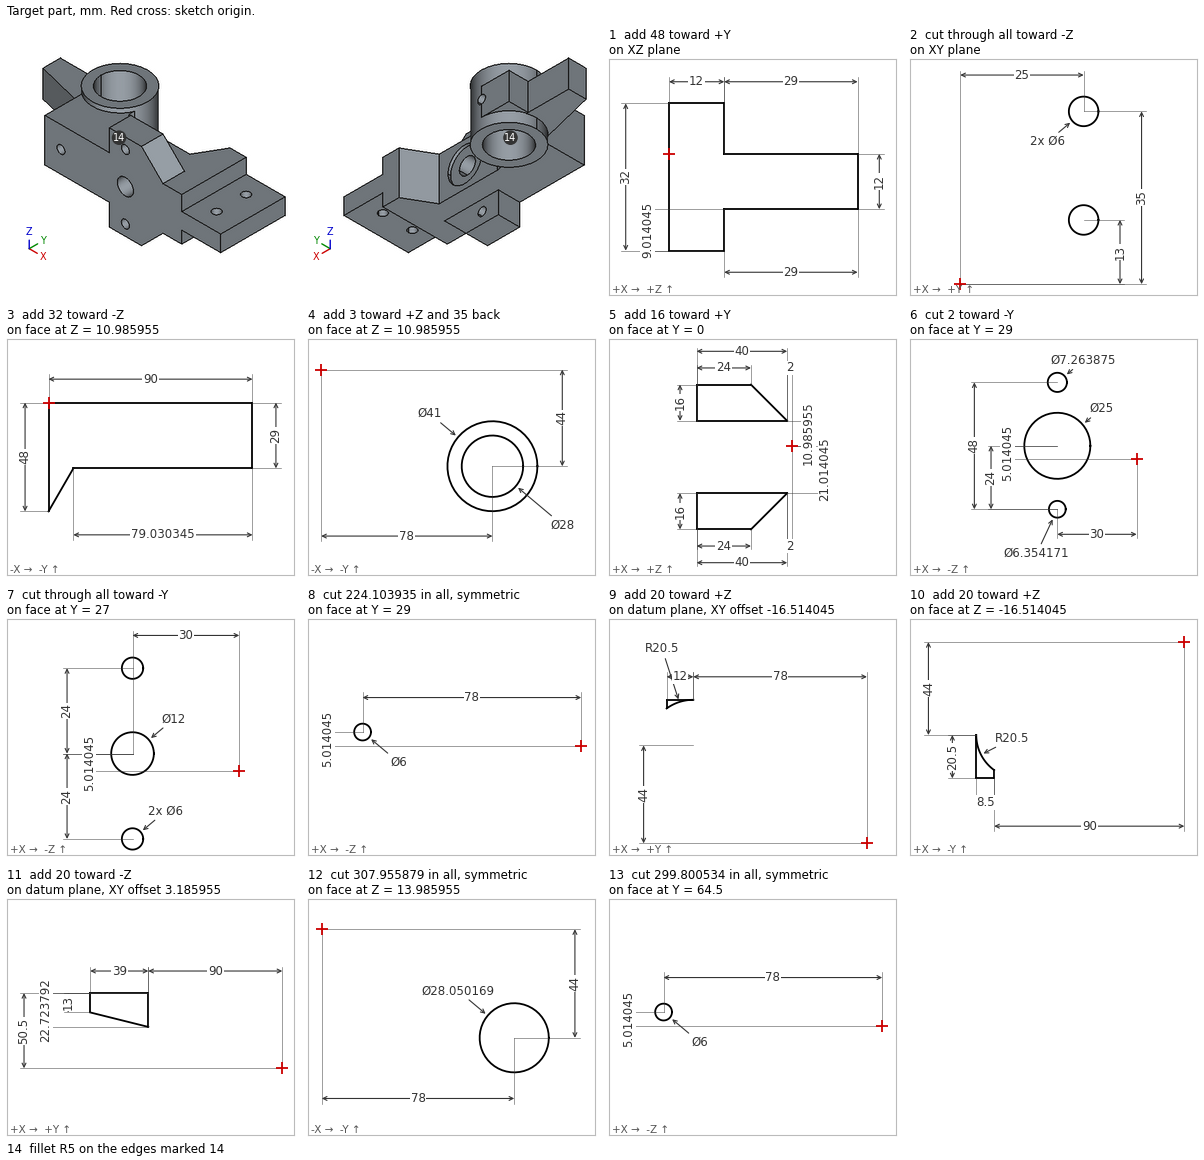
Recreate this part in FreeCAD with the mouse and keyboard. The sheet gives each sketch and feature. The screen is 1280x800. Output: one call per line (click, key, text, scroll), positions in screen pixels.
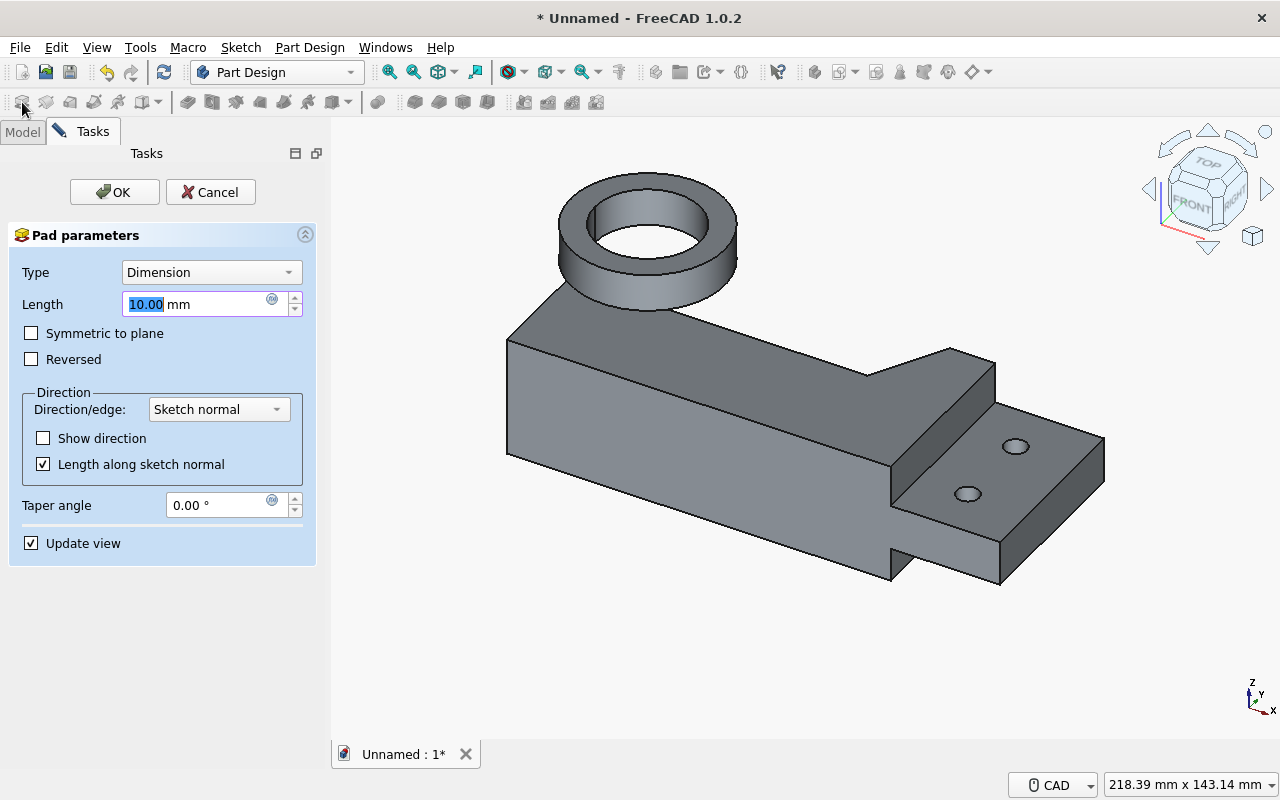
click(212, 272)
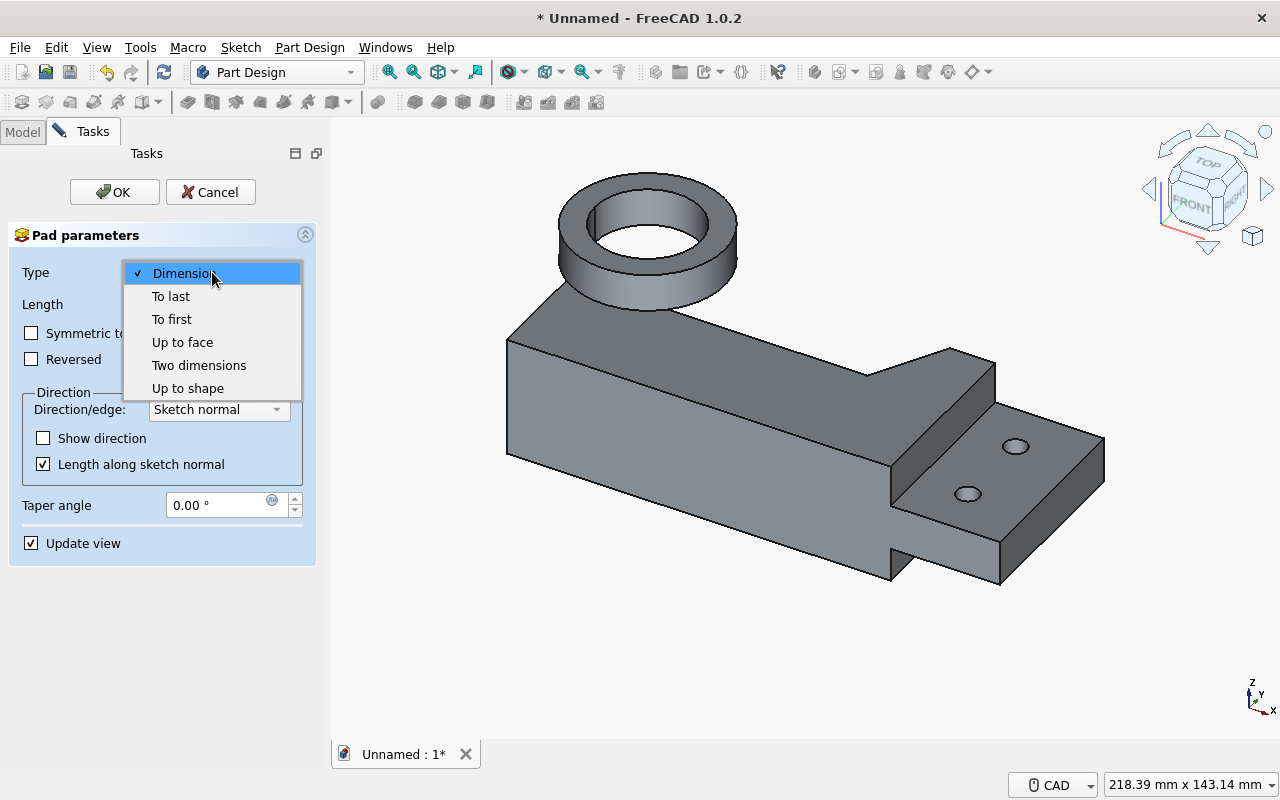
click(212, 366)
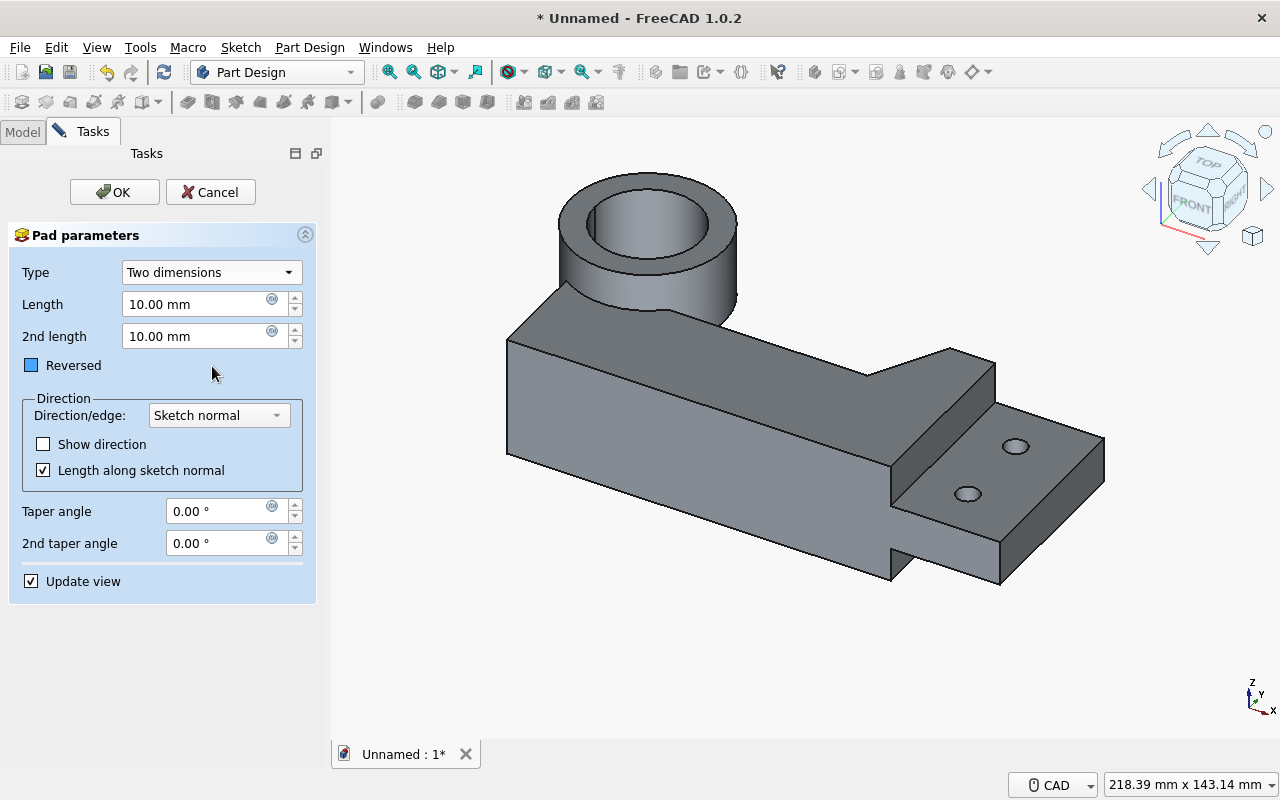
triple_click(204, 304)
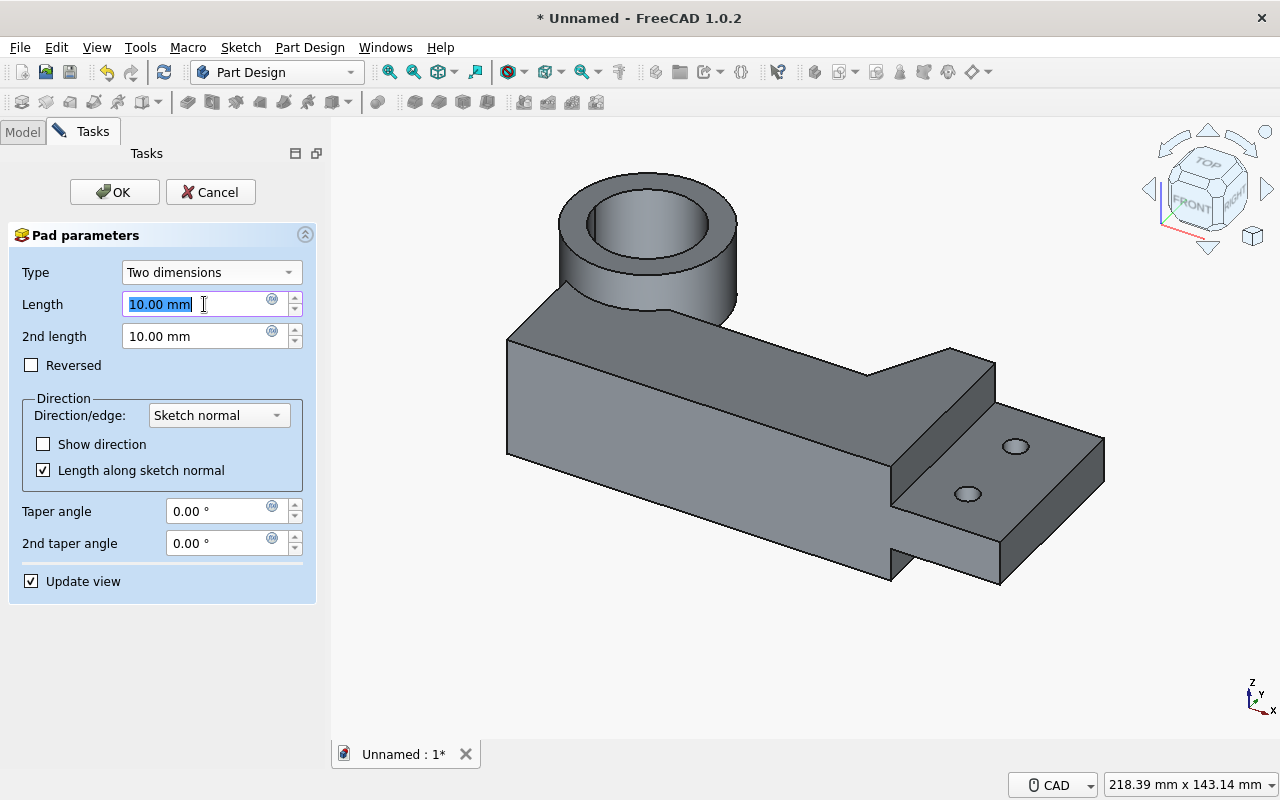
text(3)
key(Tab)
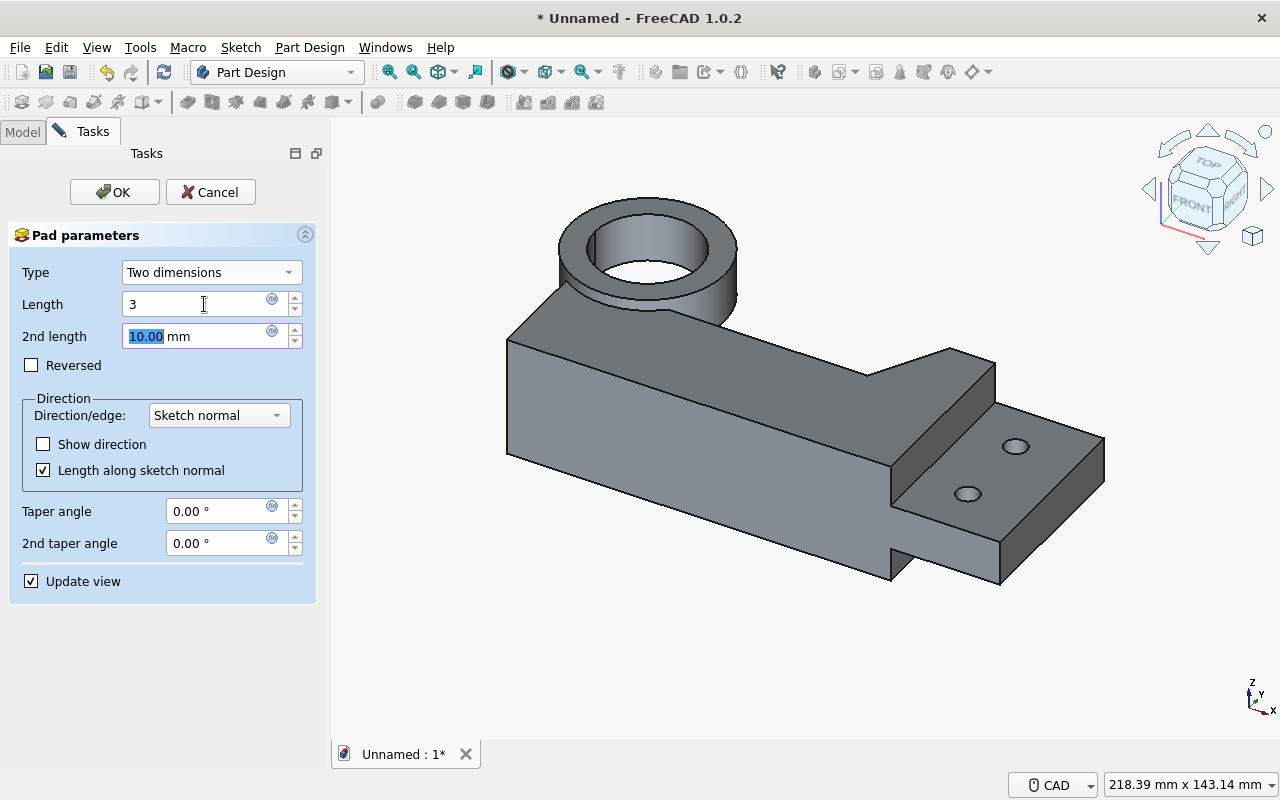
text(35)
key(Tab)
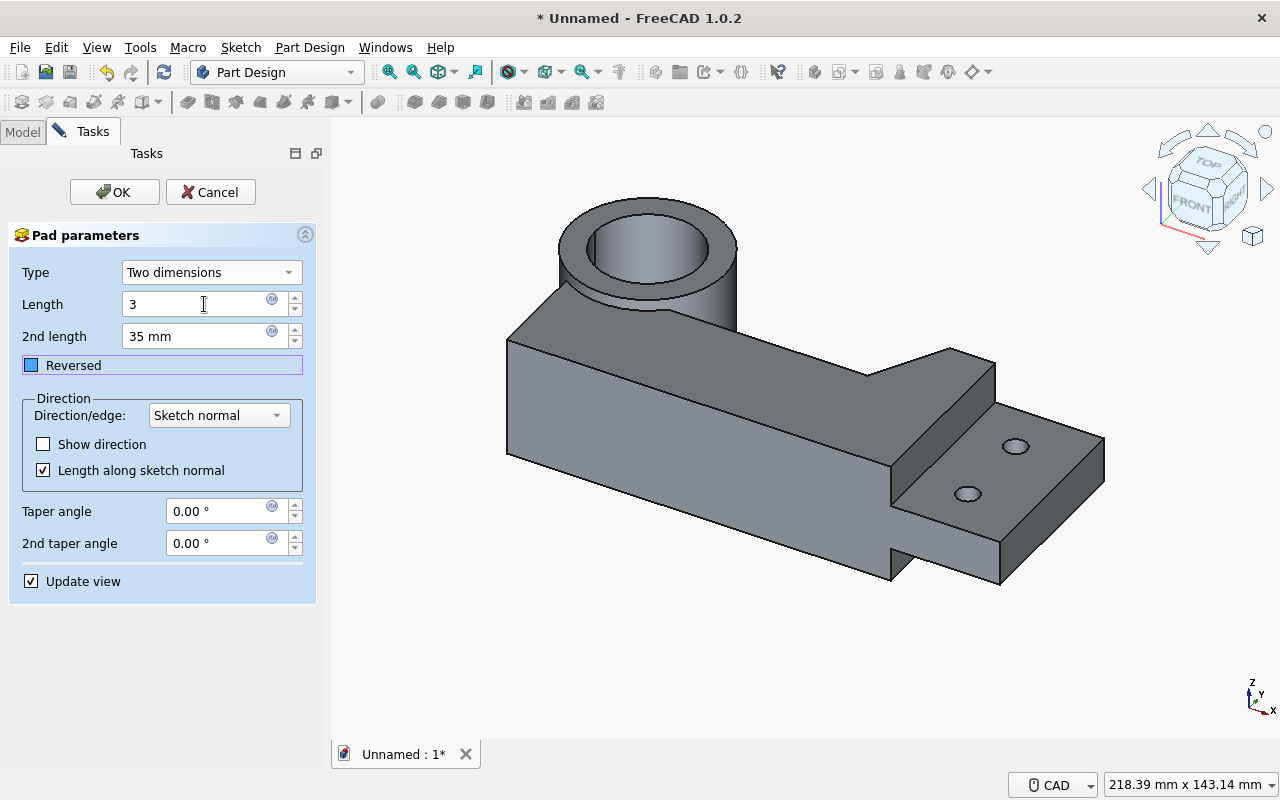
click(115, 192)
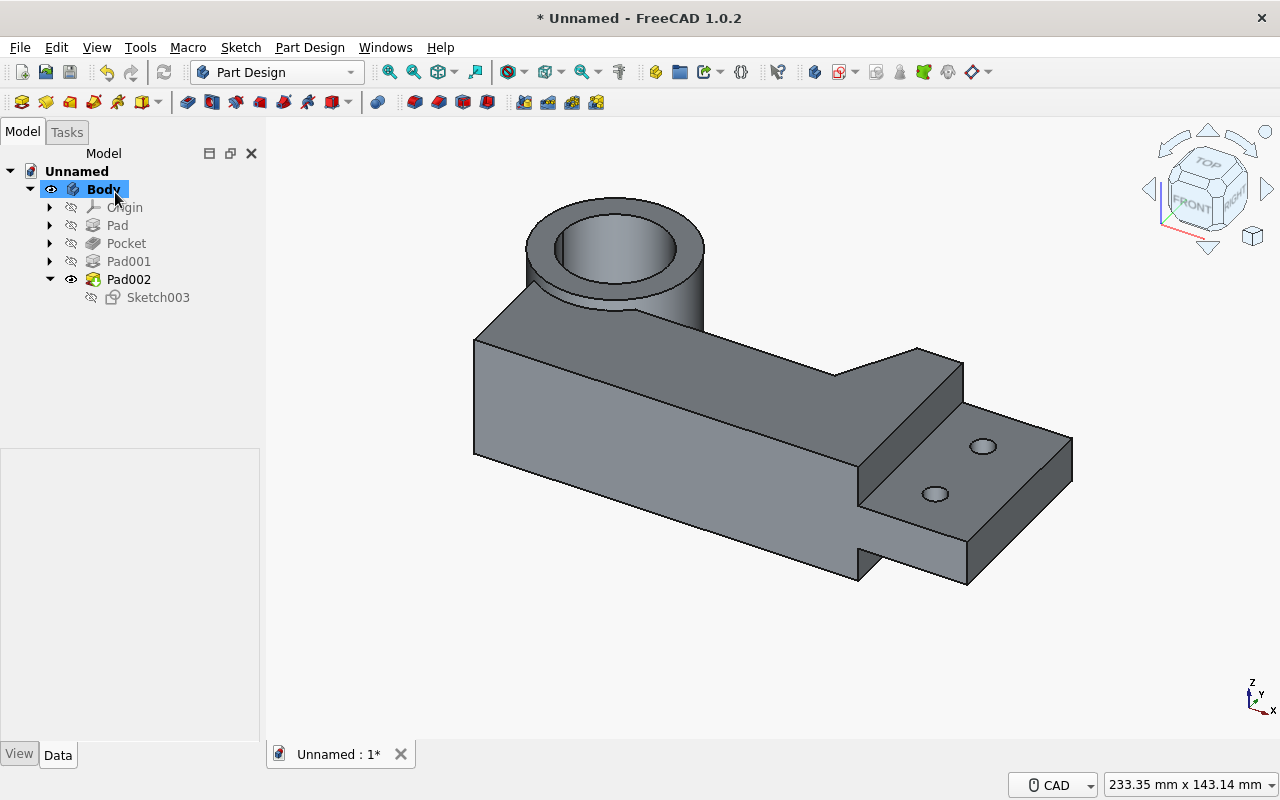
click(791, 501)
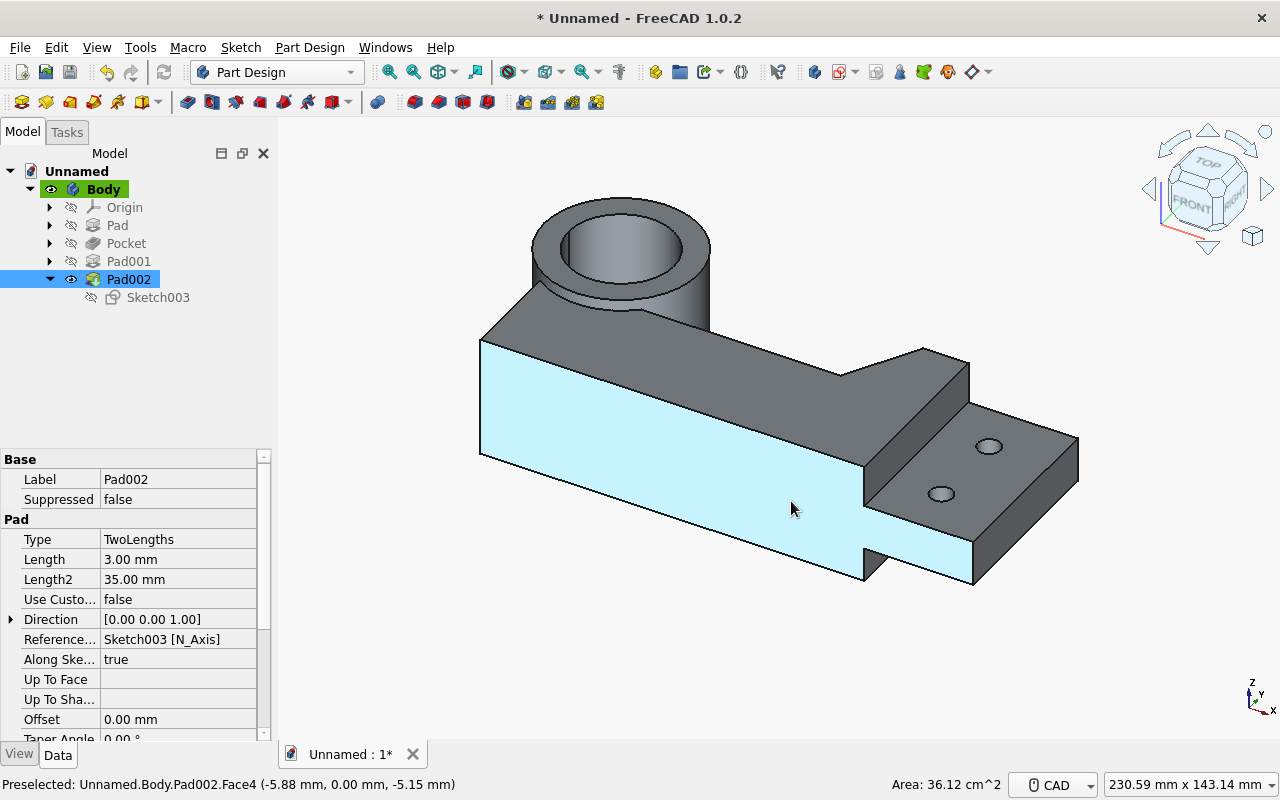
click(840, 72)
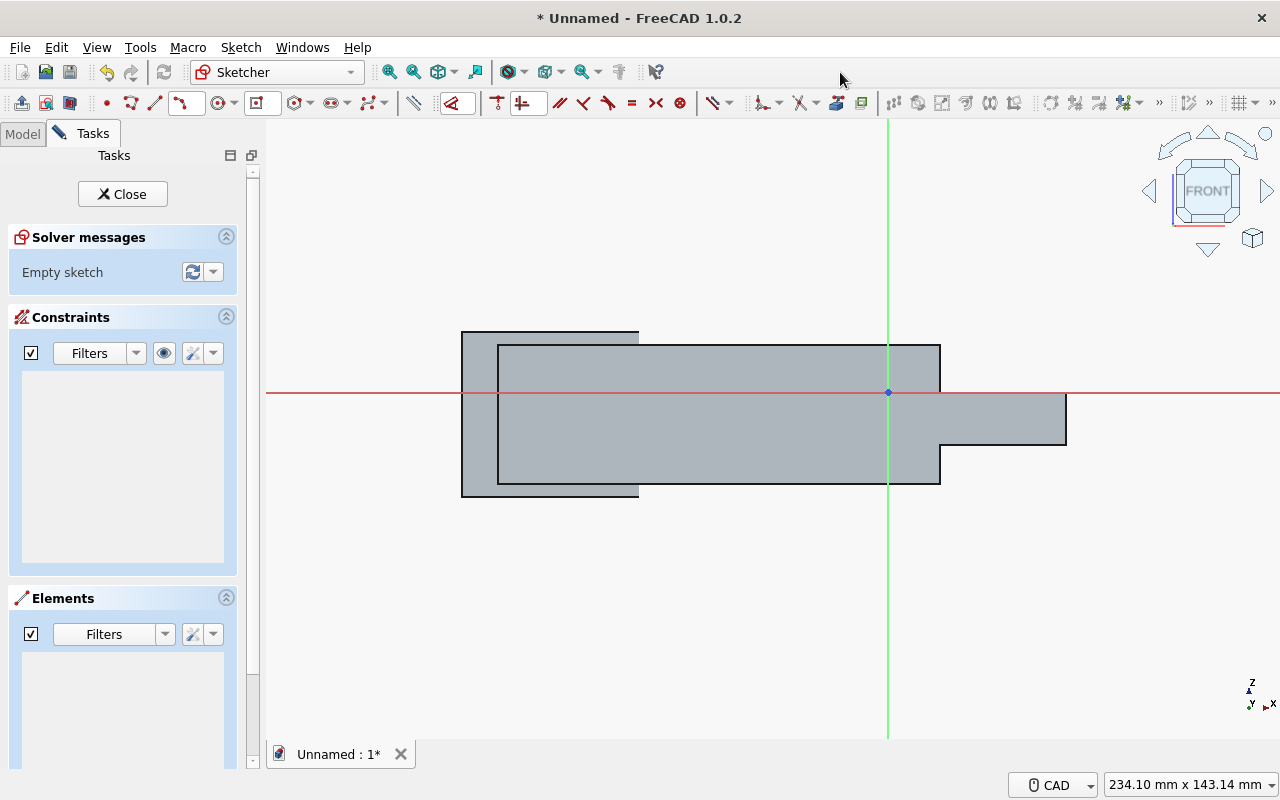
scroll(986, 385, up, 2)